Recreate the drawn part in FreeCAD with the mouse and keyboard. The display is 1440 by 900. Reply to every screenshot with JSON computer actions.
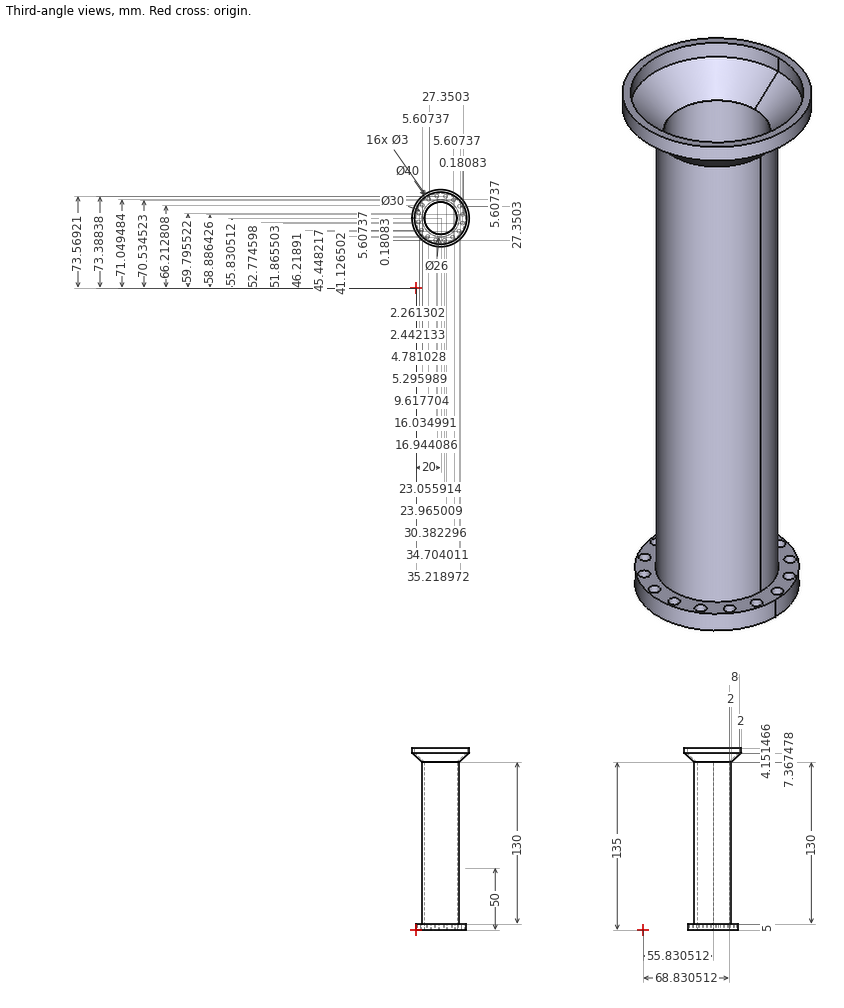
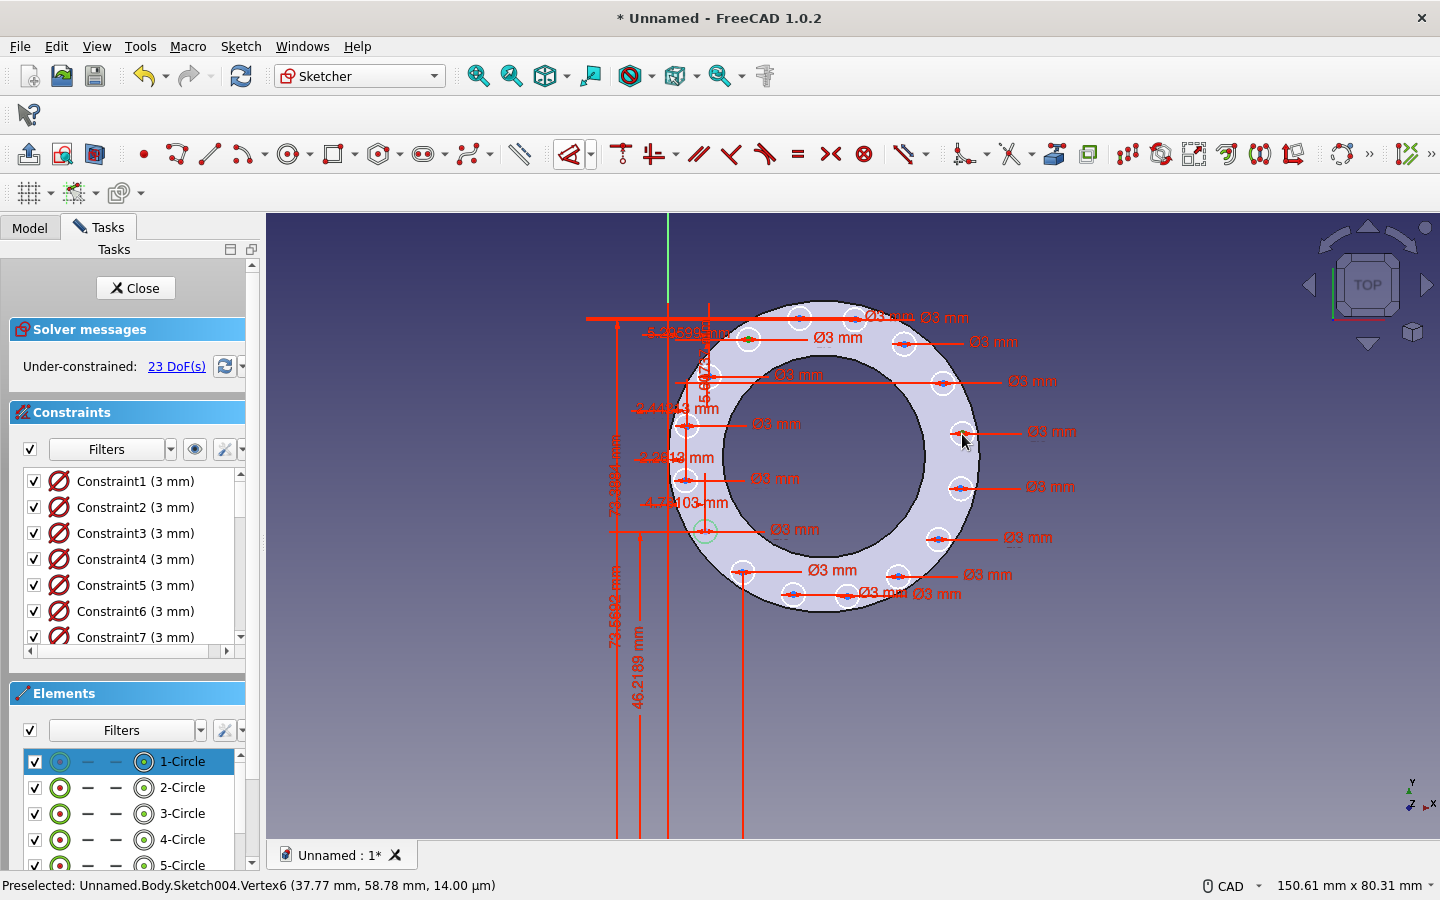
{"action": "key", "text": "l"}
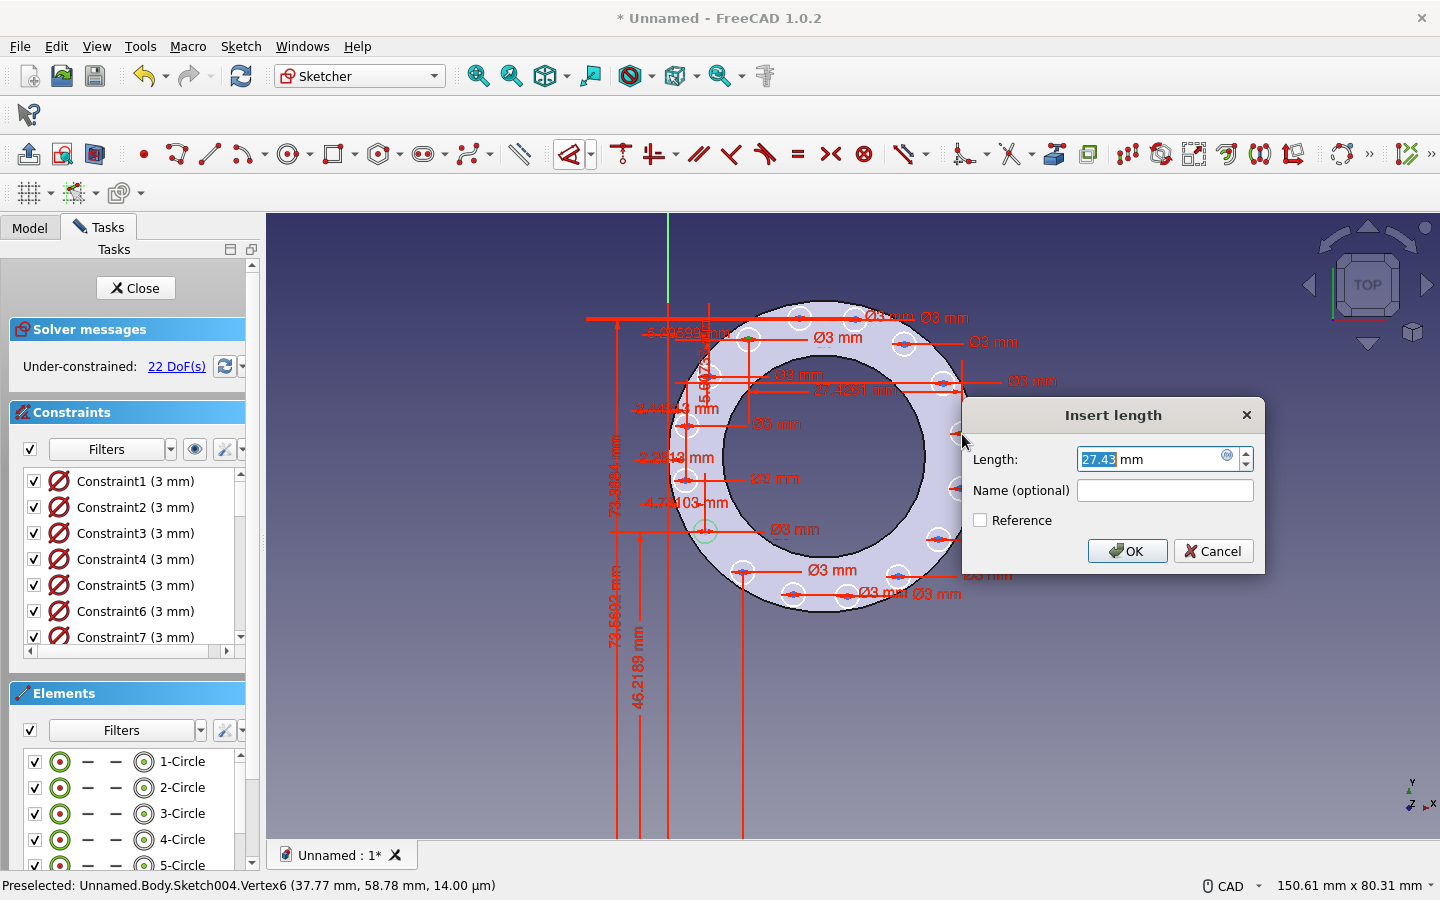
{"action": "type", "text": "27.3503"}
{"action": "key", "text": "Return"}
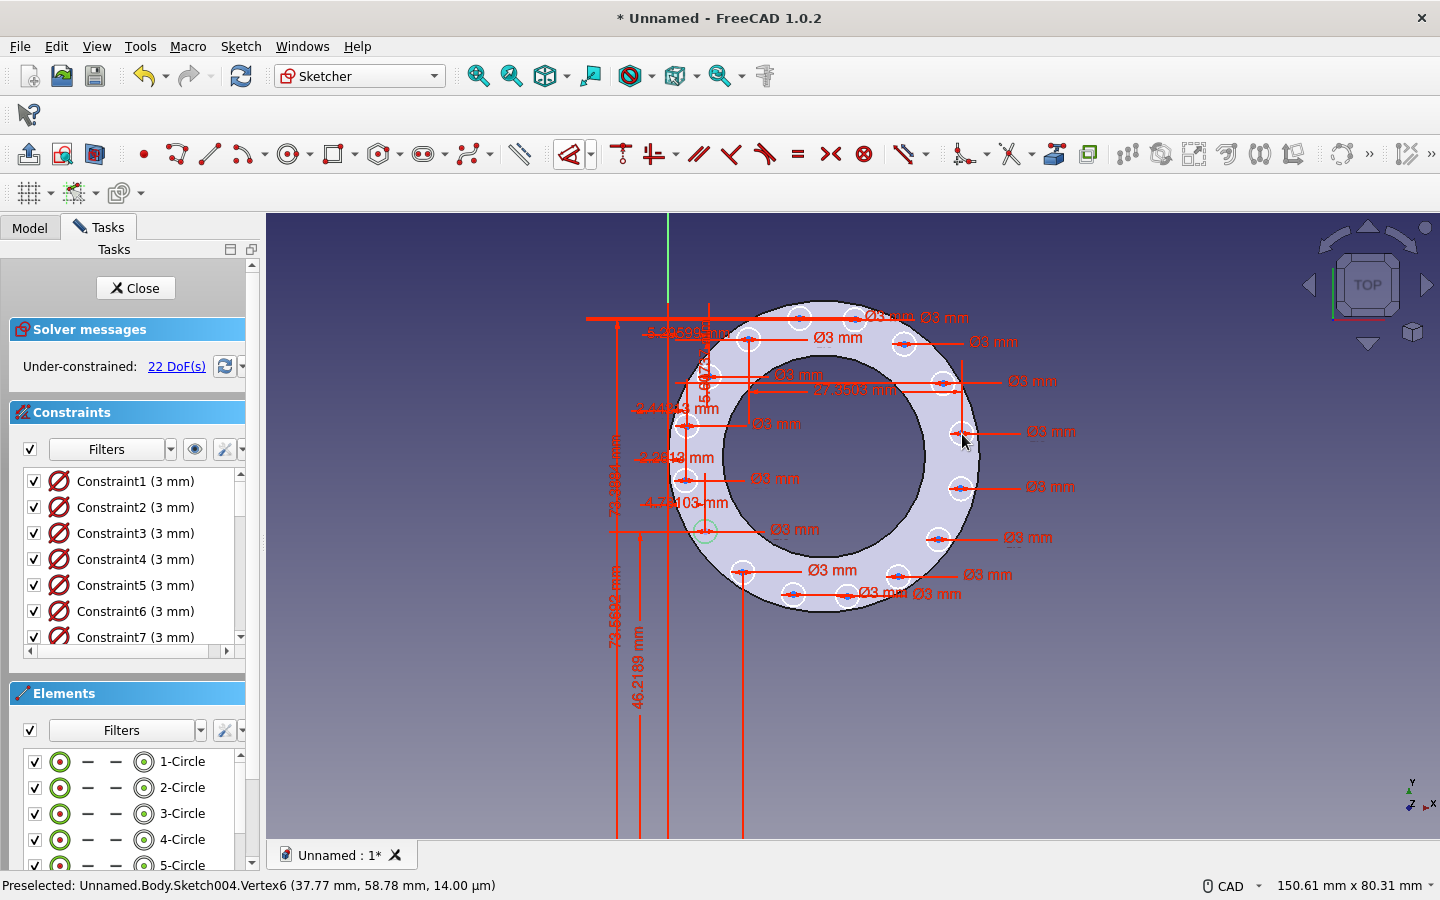
{"action": "scroll", "coordinate": [962, 434], "scroll_direction": "up", "scroll_amount": 17}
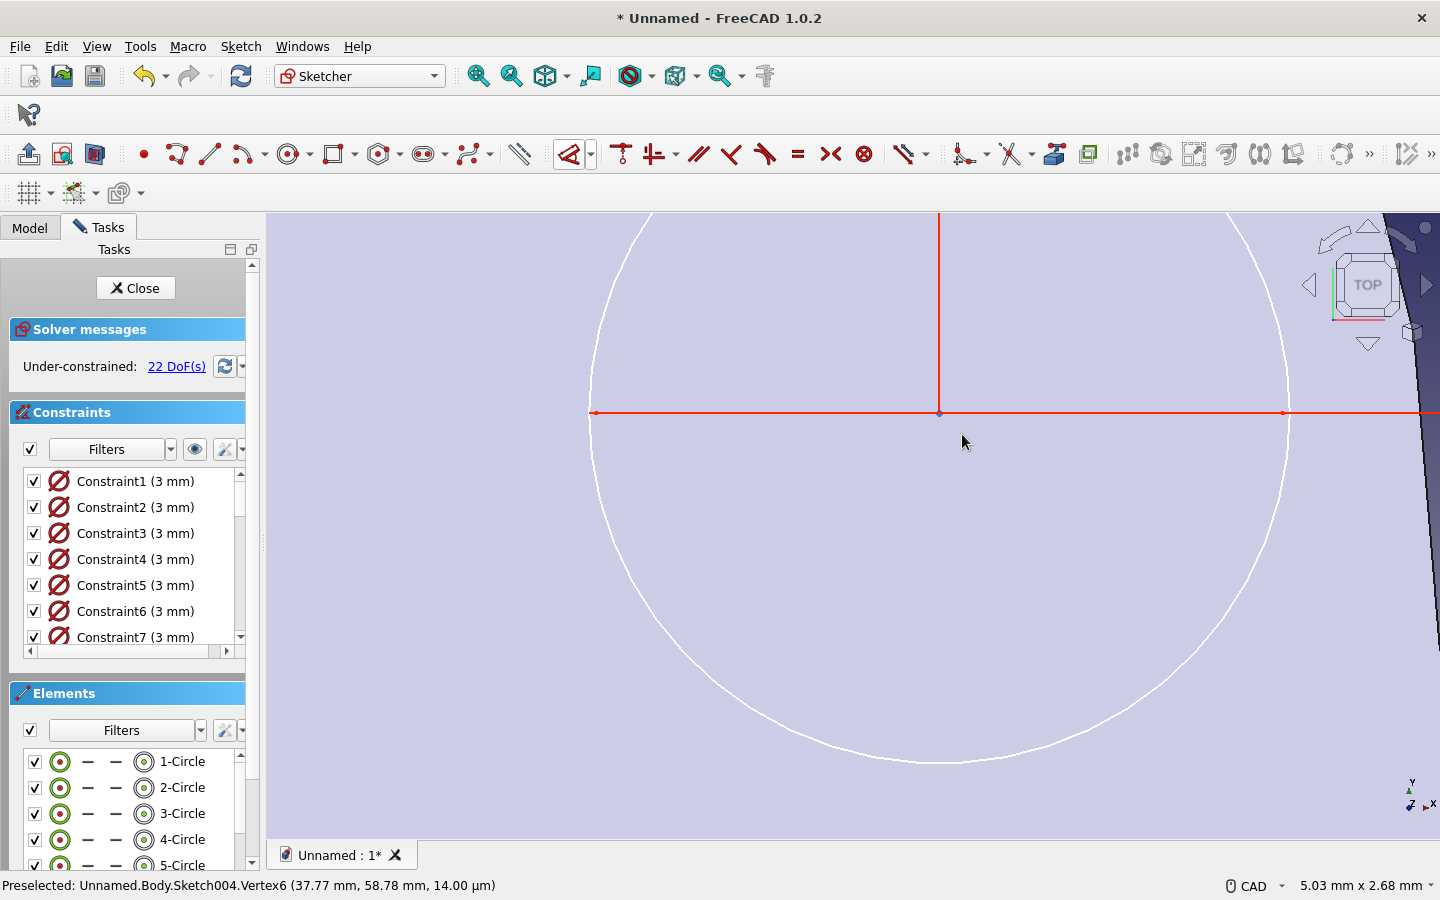
{"action": "left_click", "coordinate": [939, 413]}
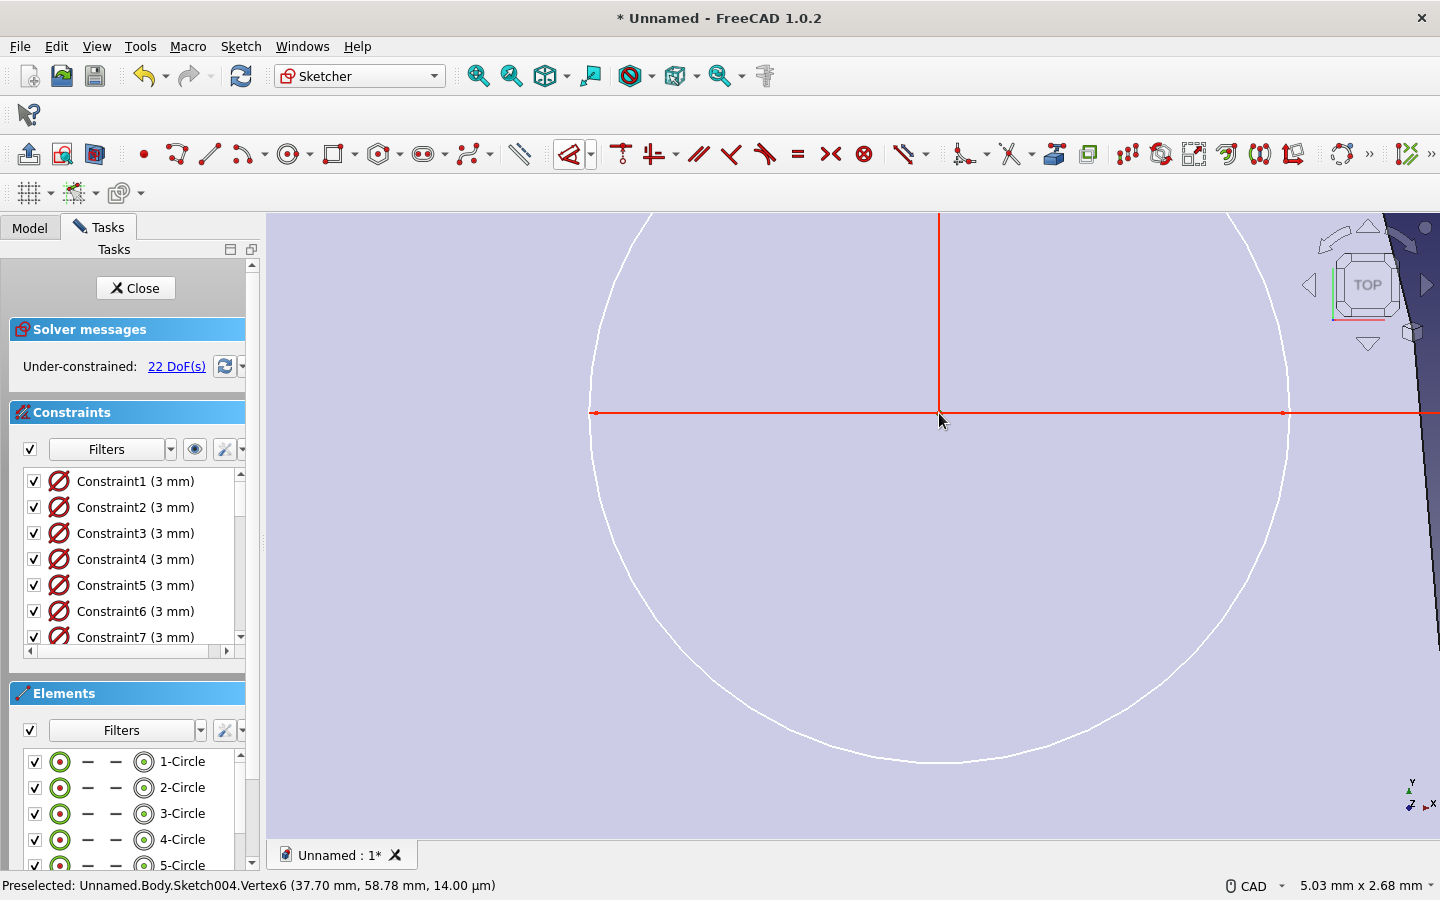
{"action": "scroll", "coordinate": [899, 390], "scroll_direction": "down", "scroll_amount": 18}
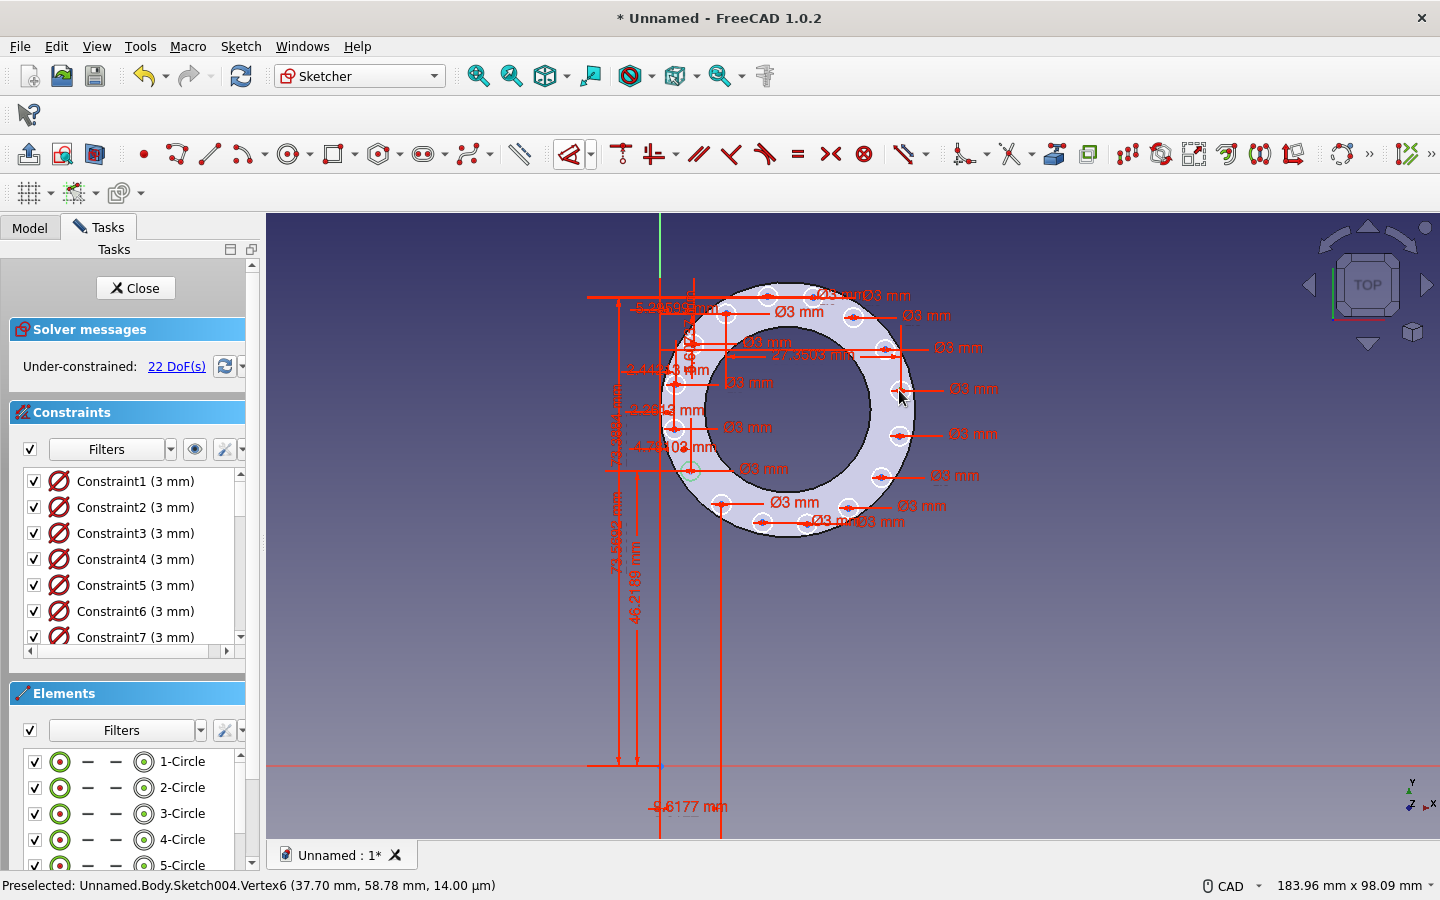
{"action": "scroll", "coordinate": [900, 436], "scroll_direction": "up", "scroll_amount": 18}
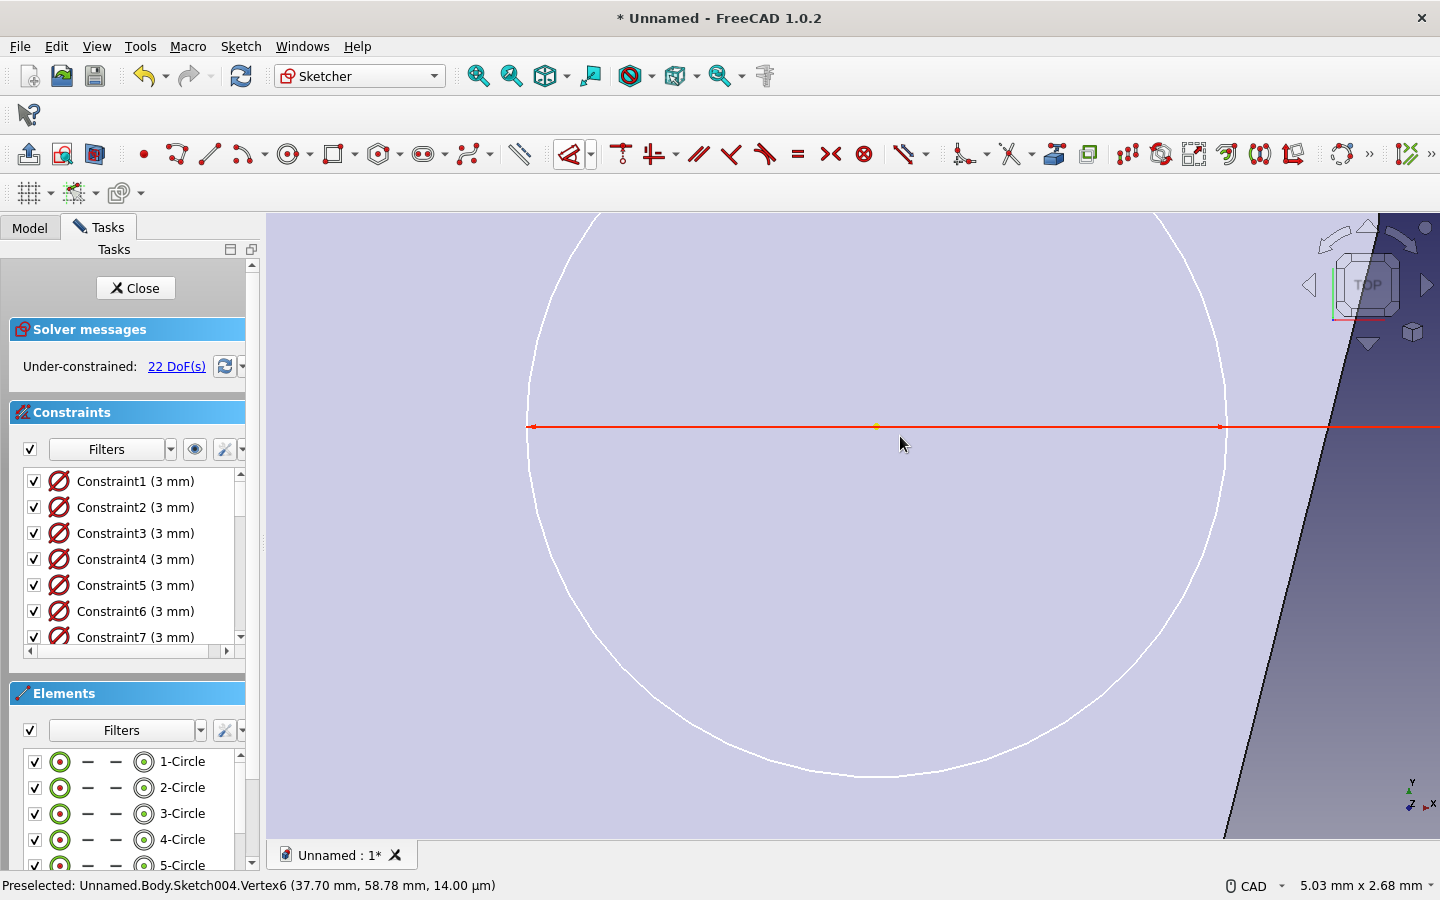
{"action": "left_click", "coordinate": [877, 427]}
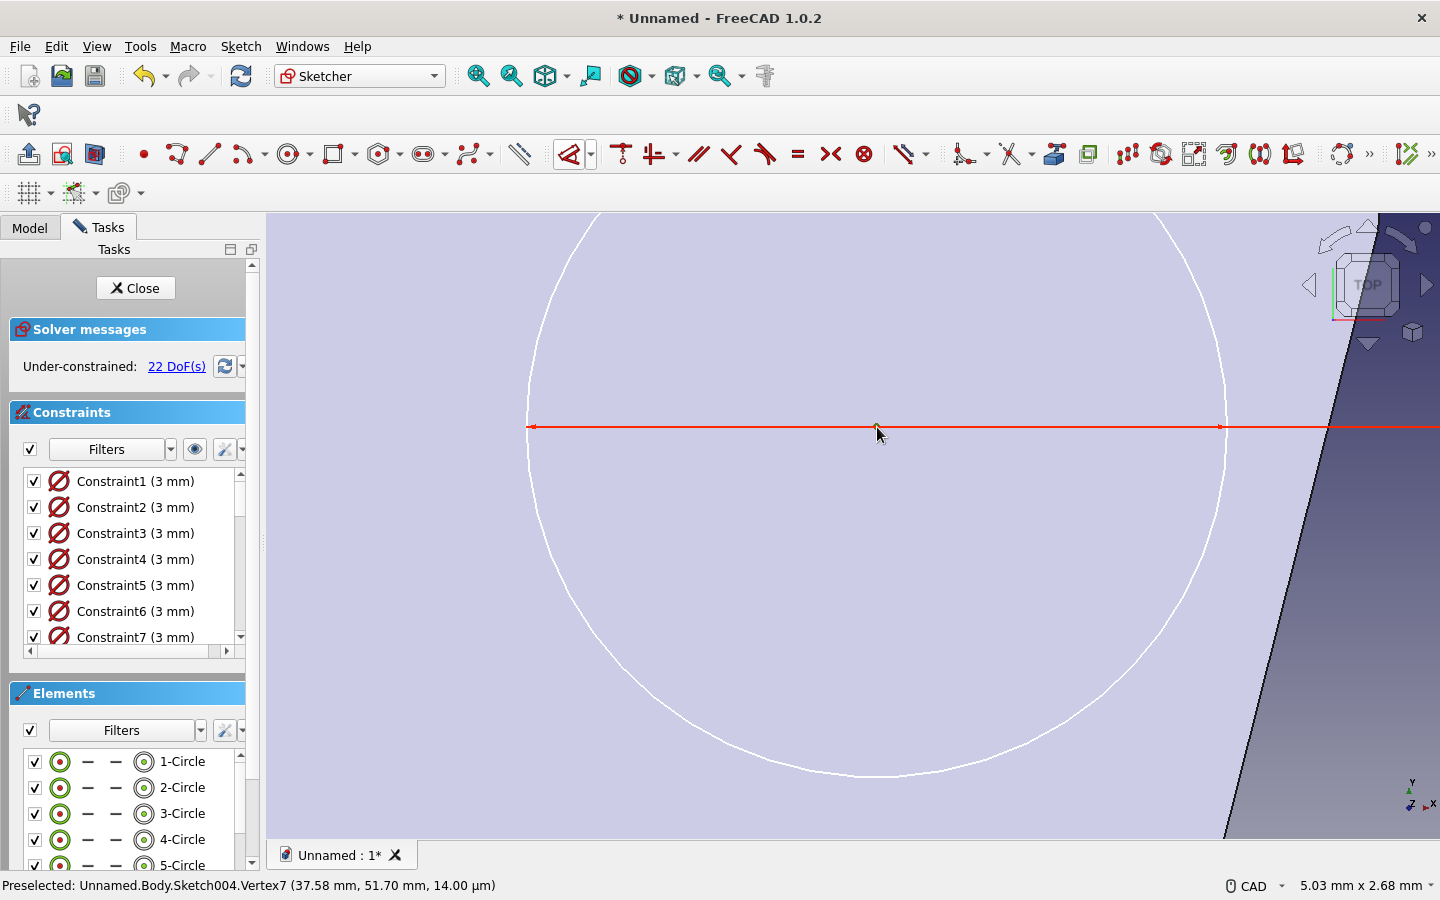
{"action": "key", "text": "l"}